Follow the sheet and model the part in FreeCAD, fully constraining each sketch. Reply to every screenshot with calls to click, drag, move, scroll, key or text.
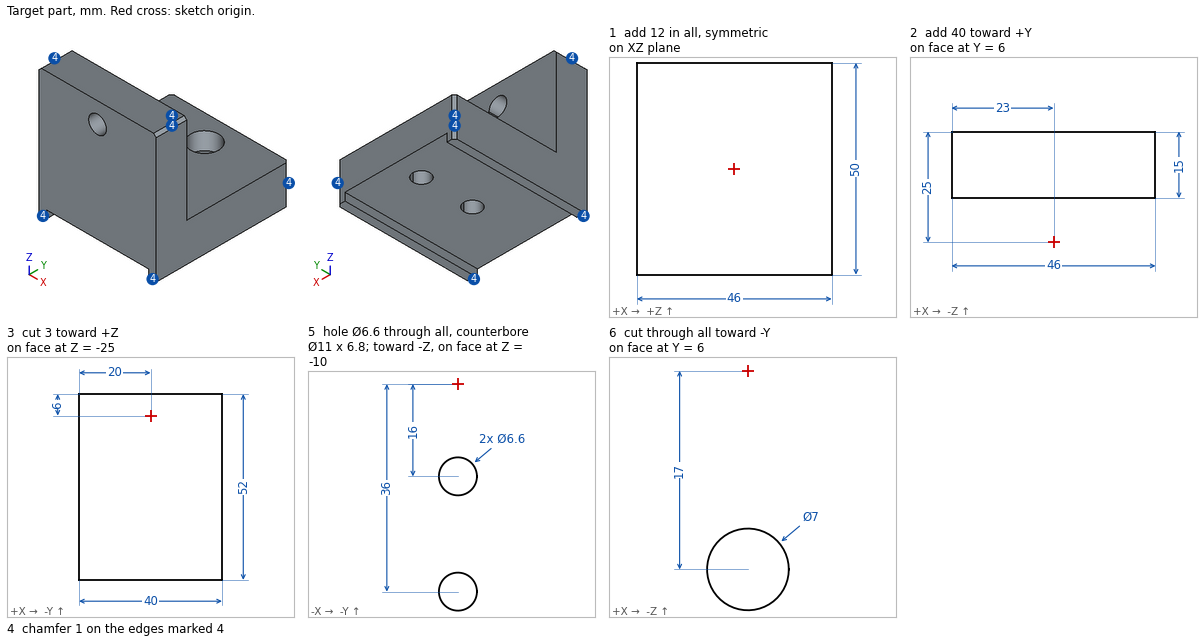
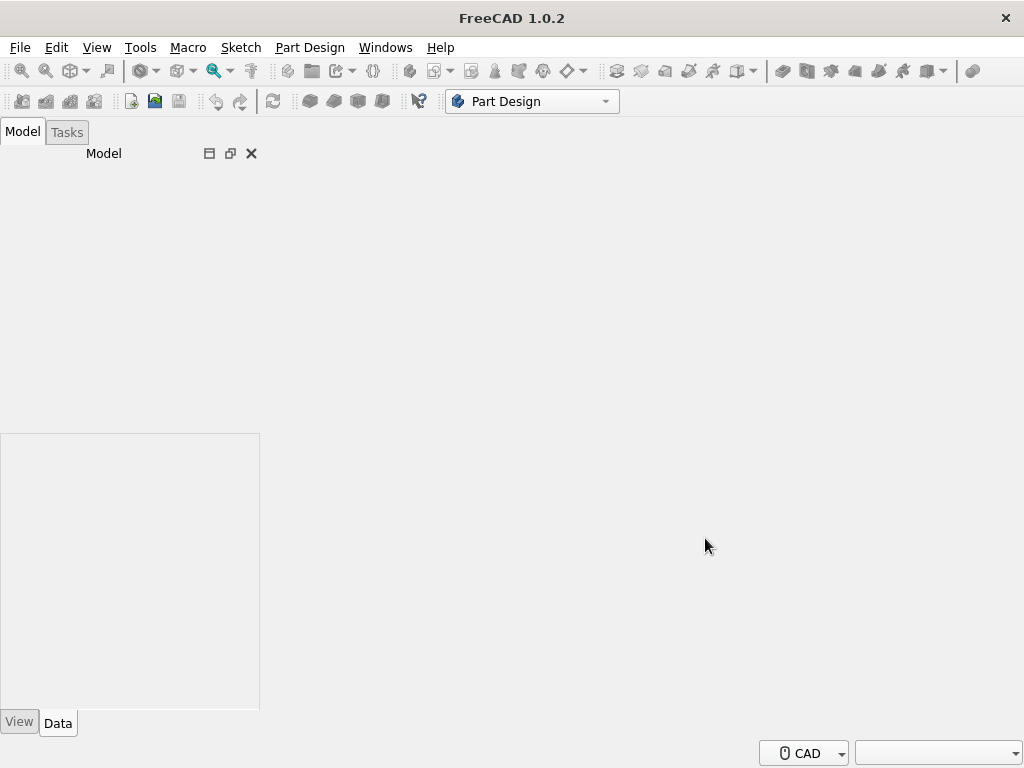
click(132, 102)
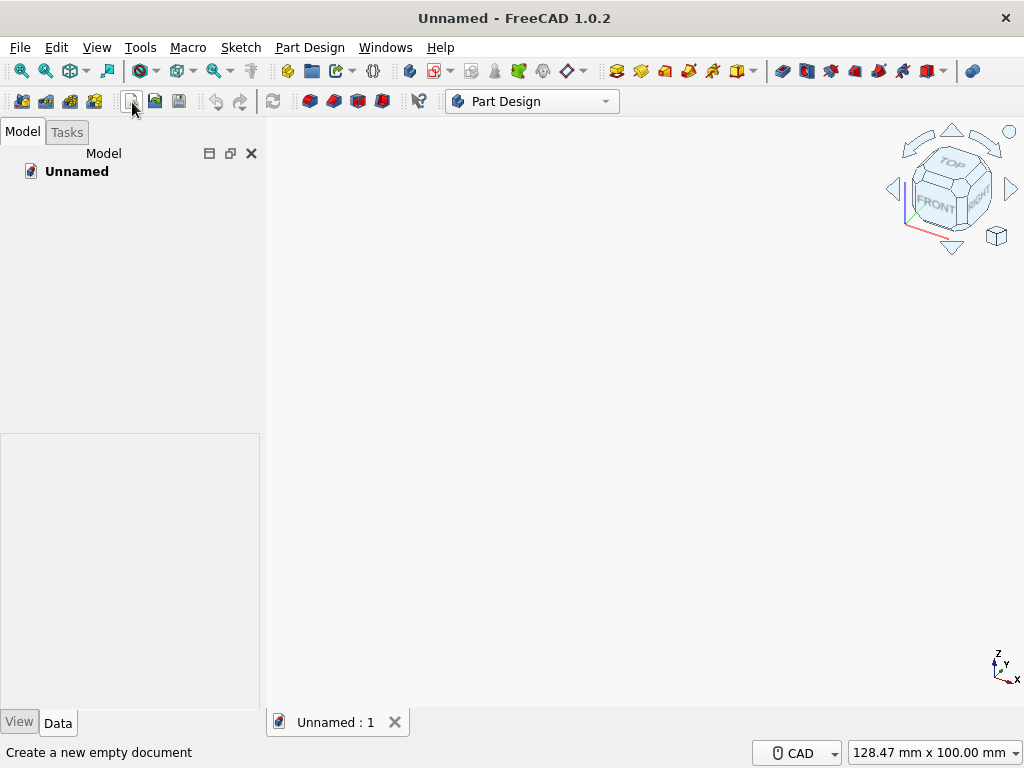
click(434, 72)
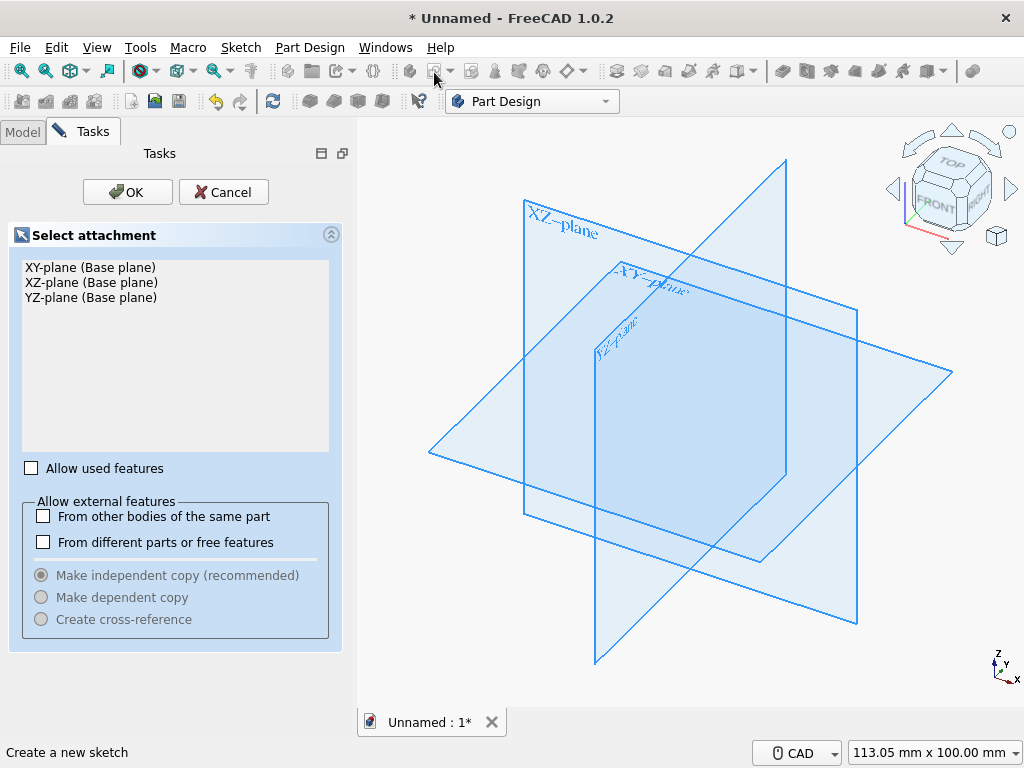
click(82, 282)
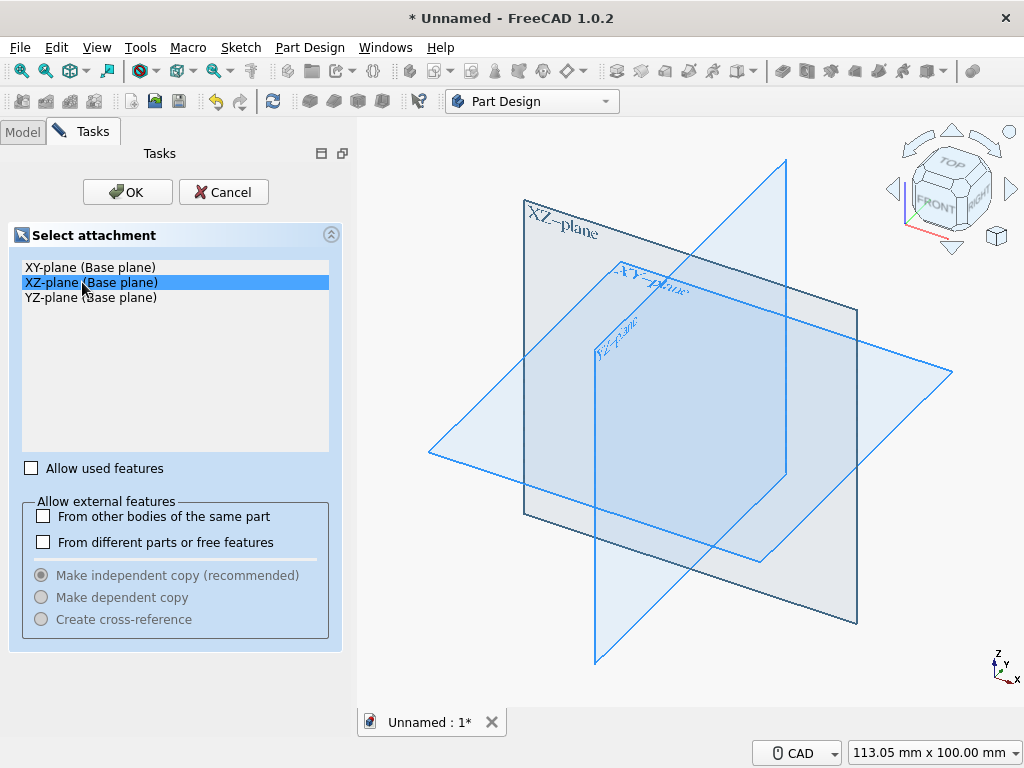
click(128, 192)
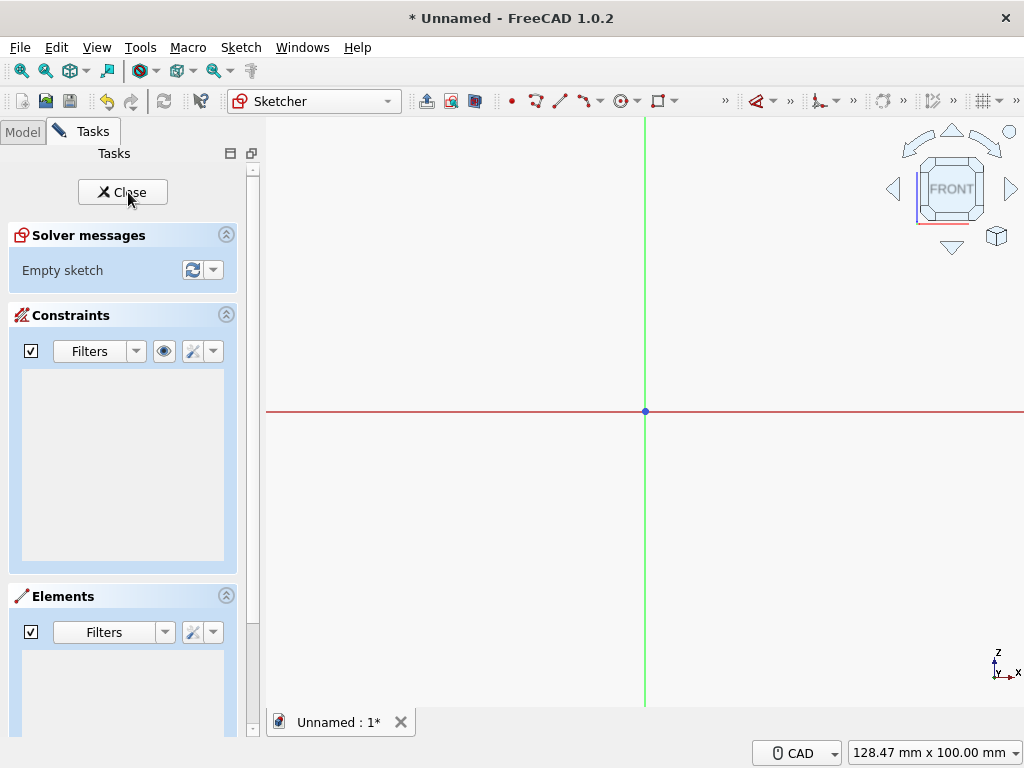
key(g)
key(v)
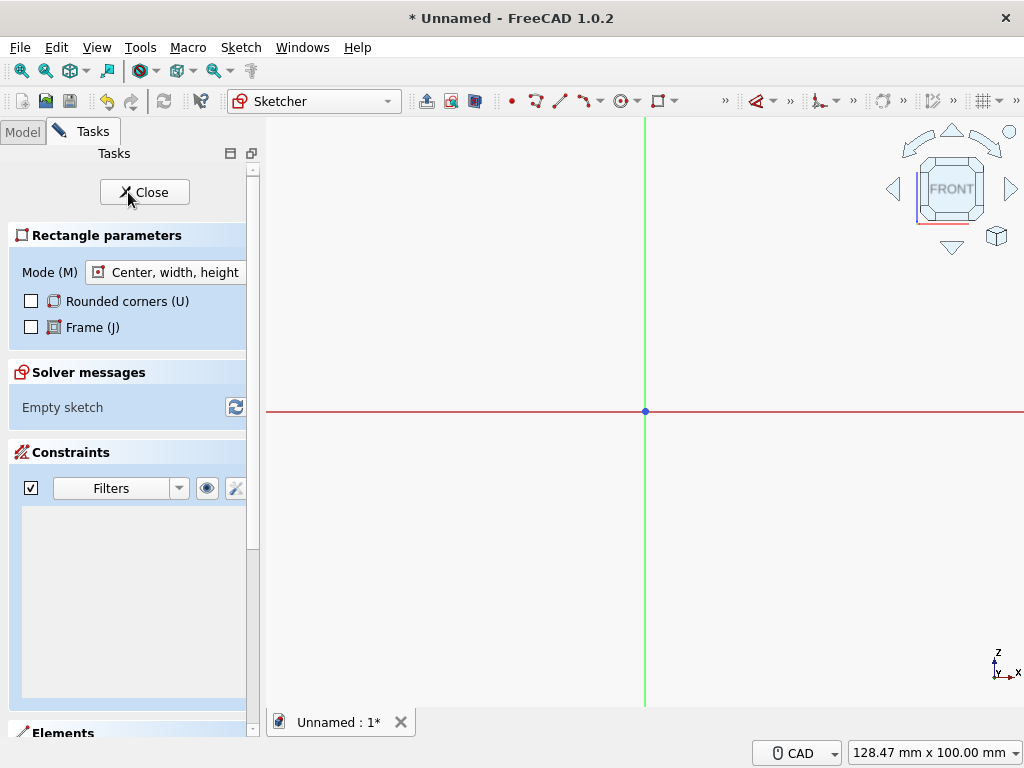
click(645, 412)
move(781, 264)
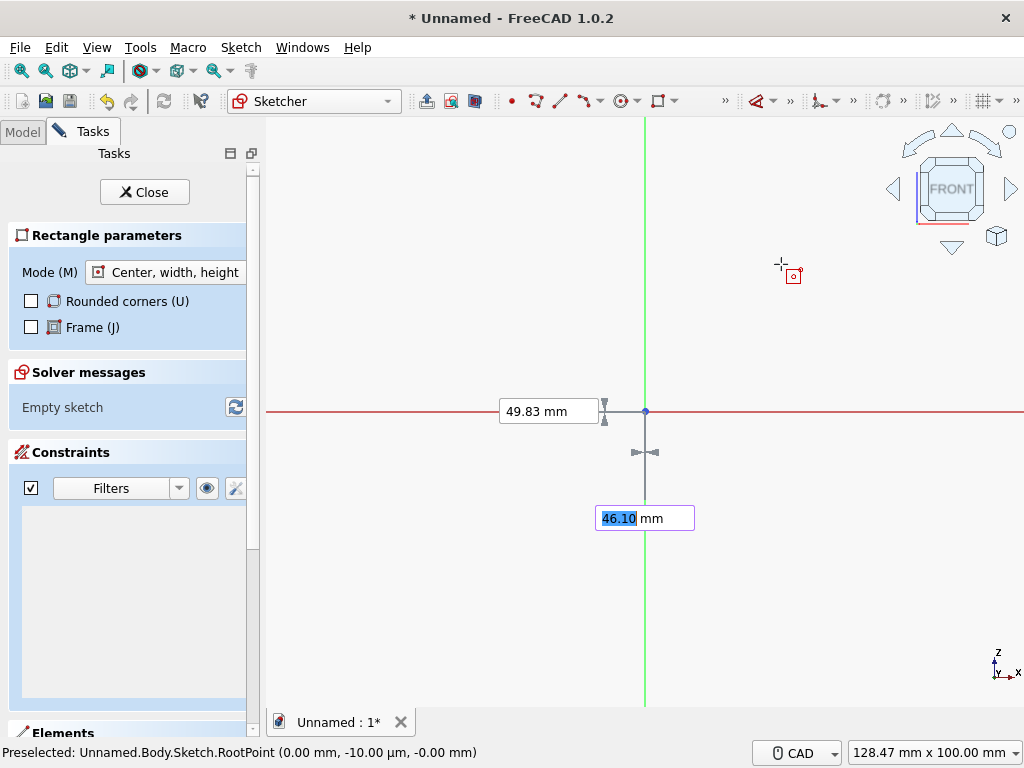
text(46)
key(Tab)
text(50)
key(Return)
key(Escape)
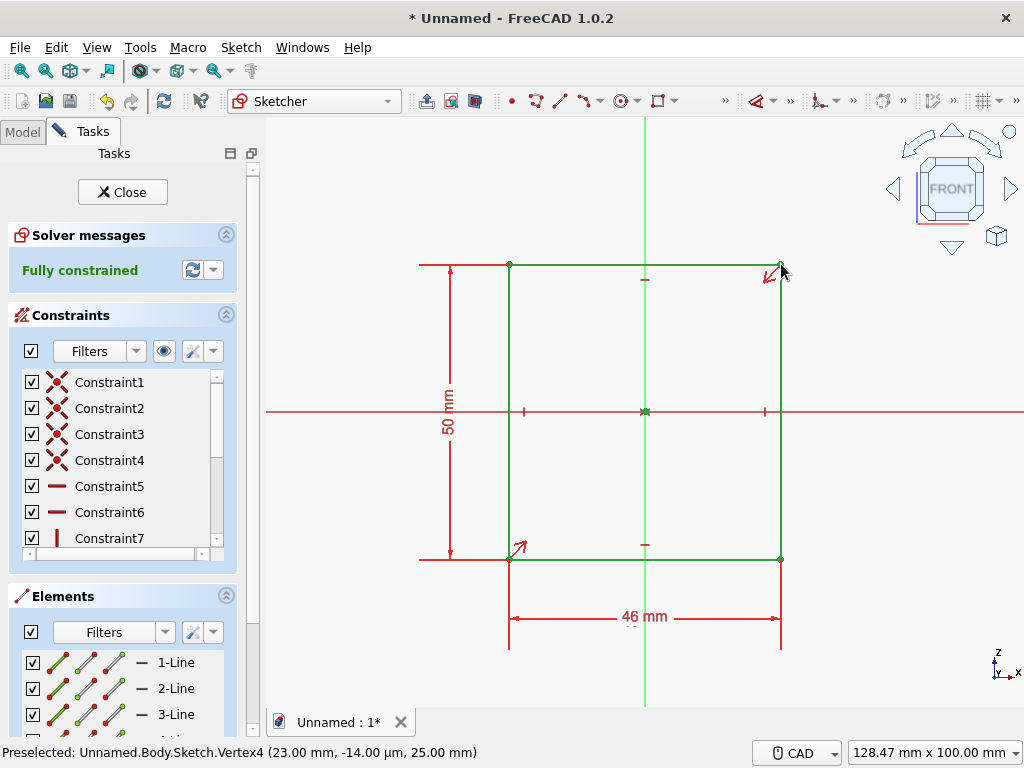
click(123, 192)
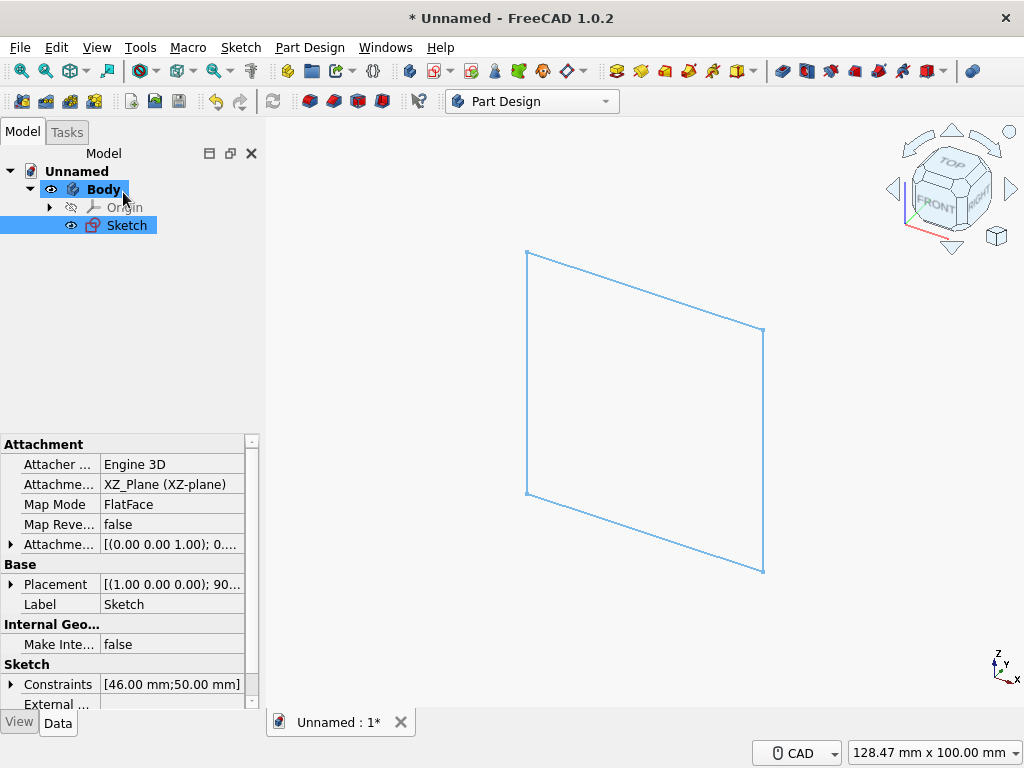
click(618, 72)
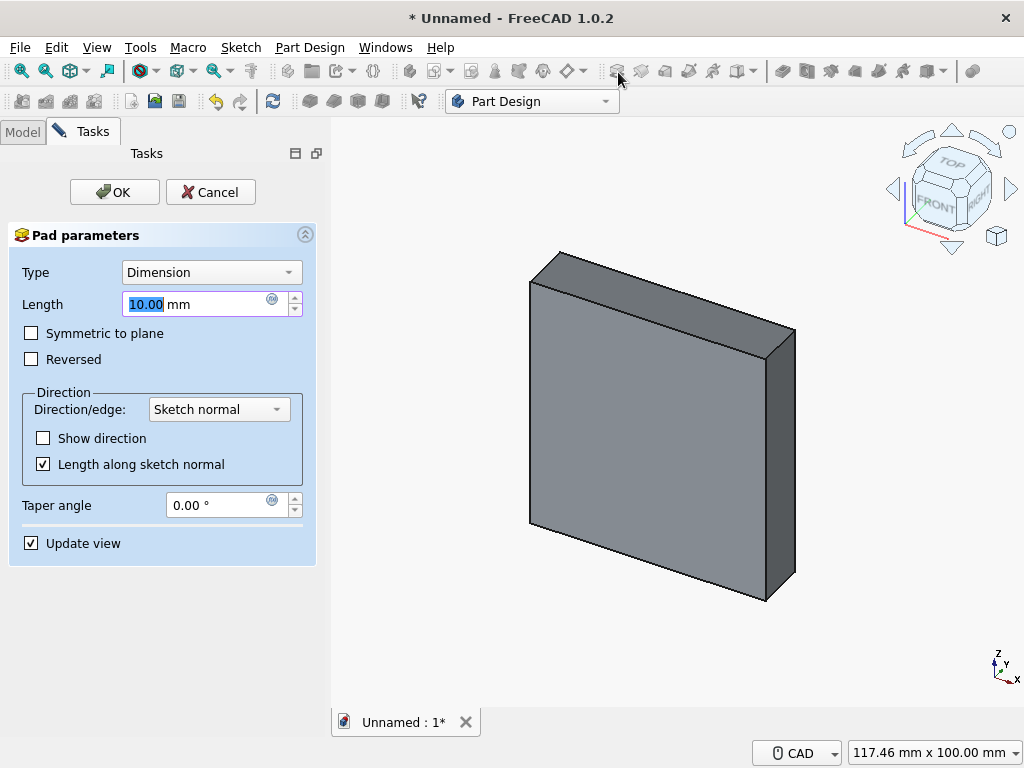
text(12)
key(Tab)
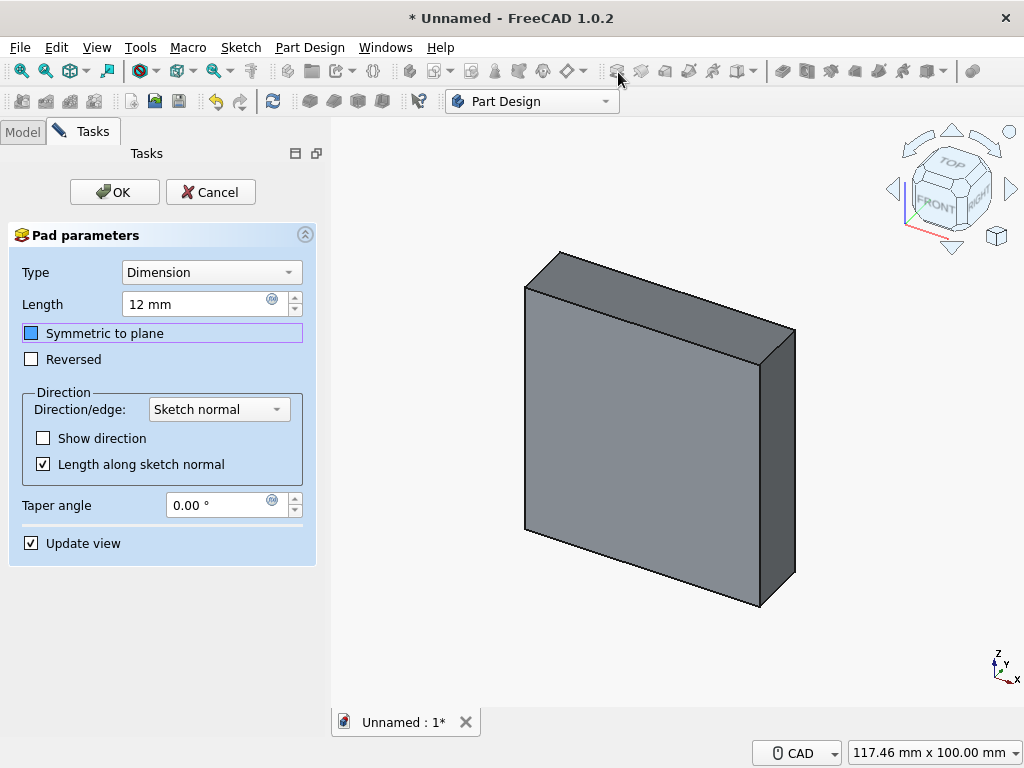
click(30, 333)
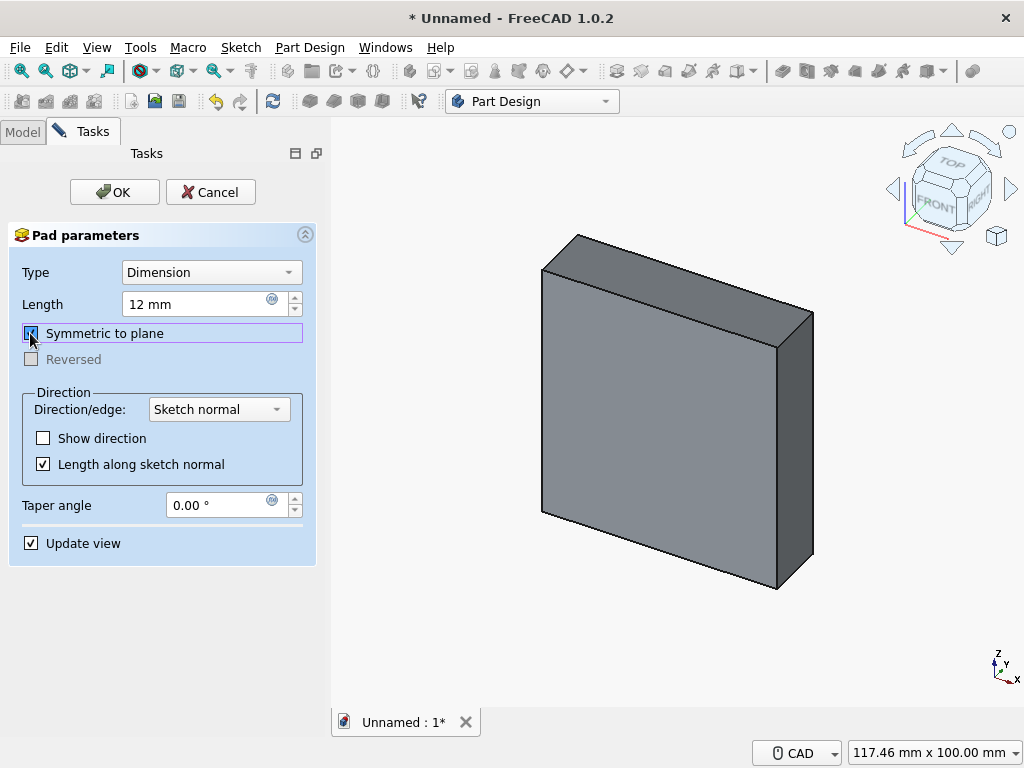
click(115, 192)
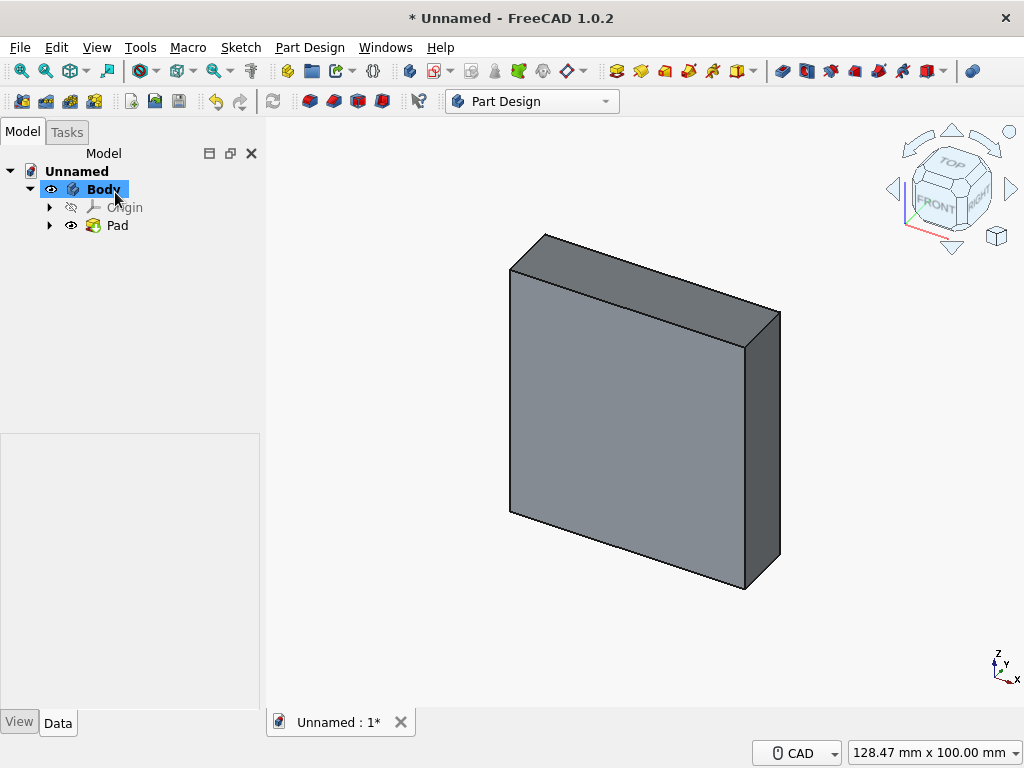
key(4)